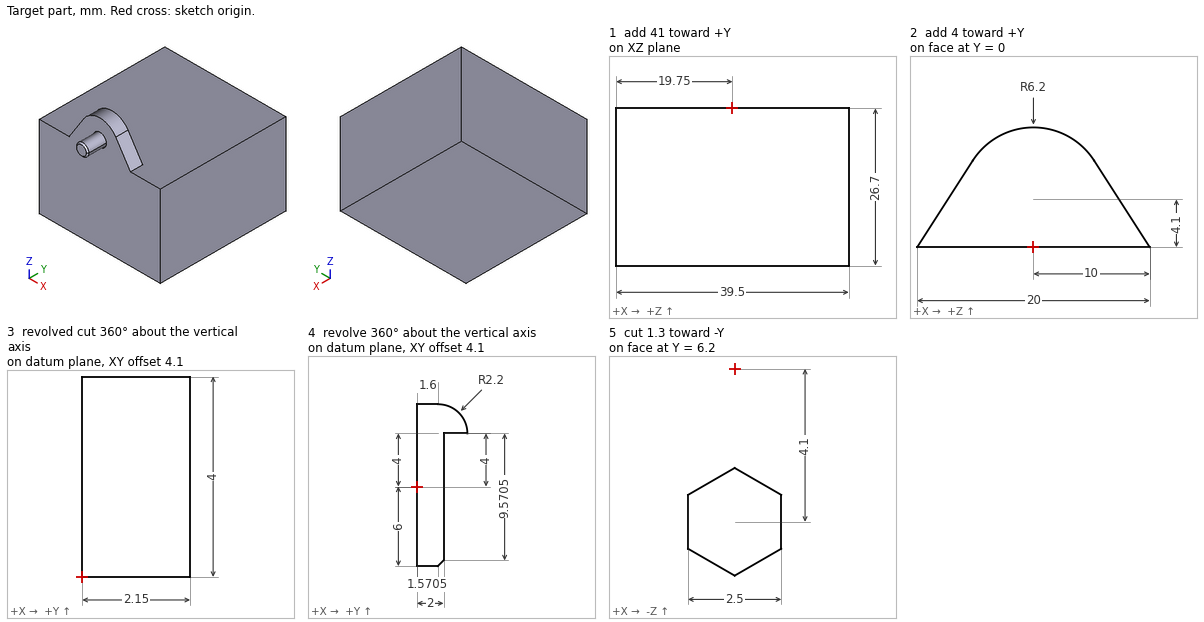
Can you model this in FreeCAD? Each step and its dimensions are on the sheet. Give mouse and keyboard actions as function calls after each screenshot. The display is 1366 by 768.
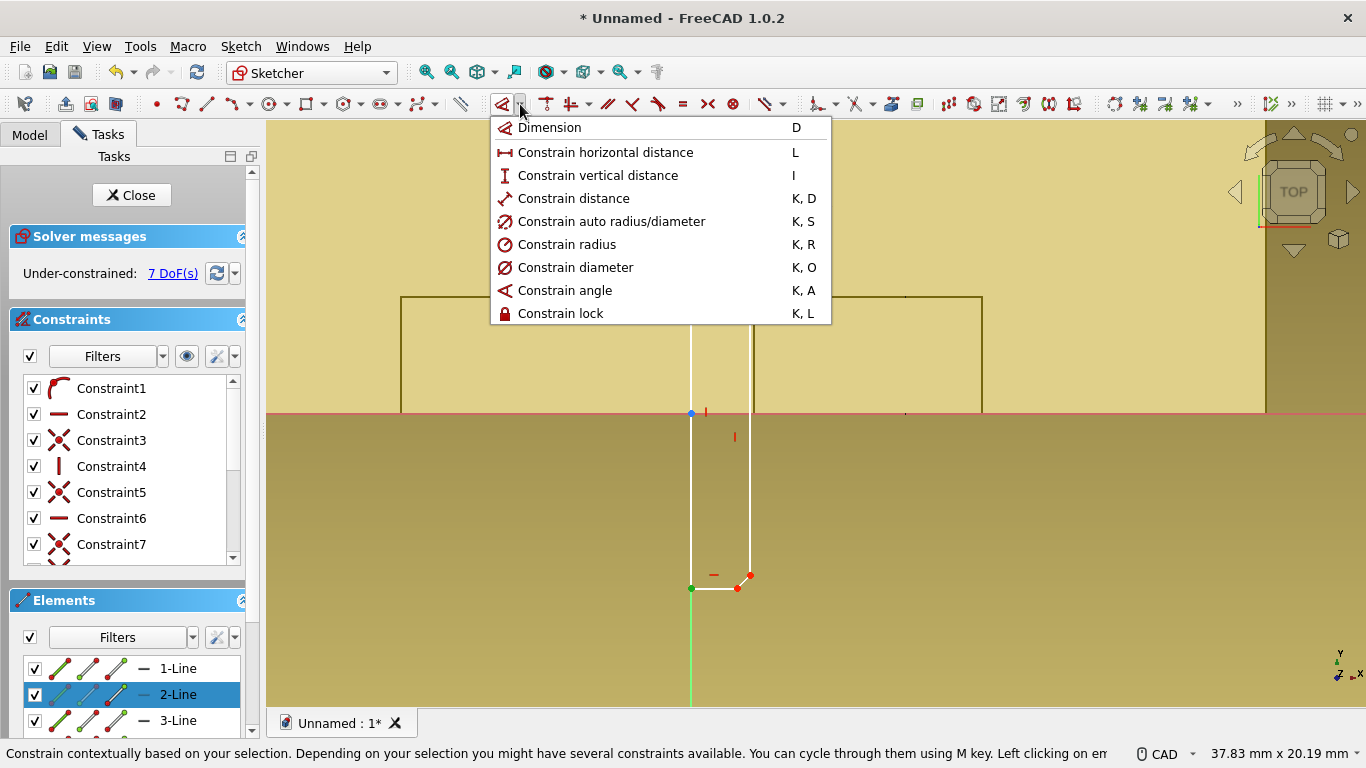
click(661, 176)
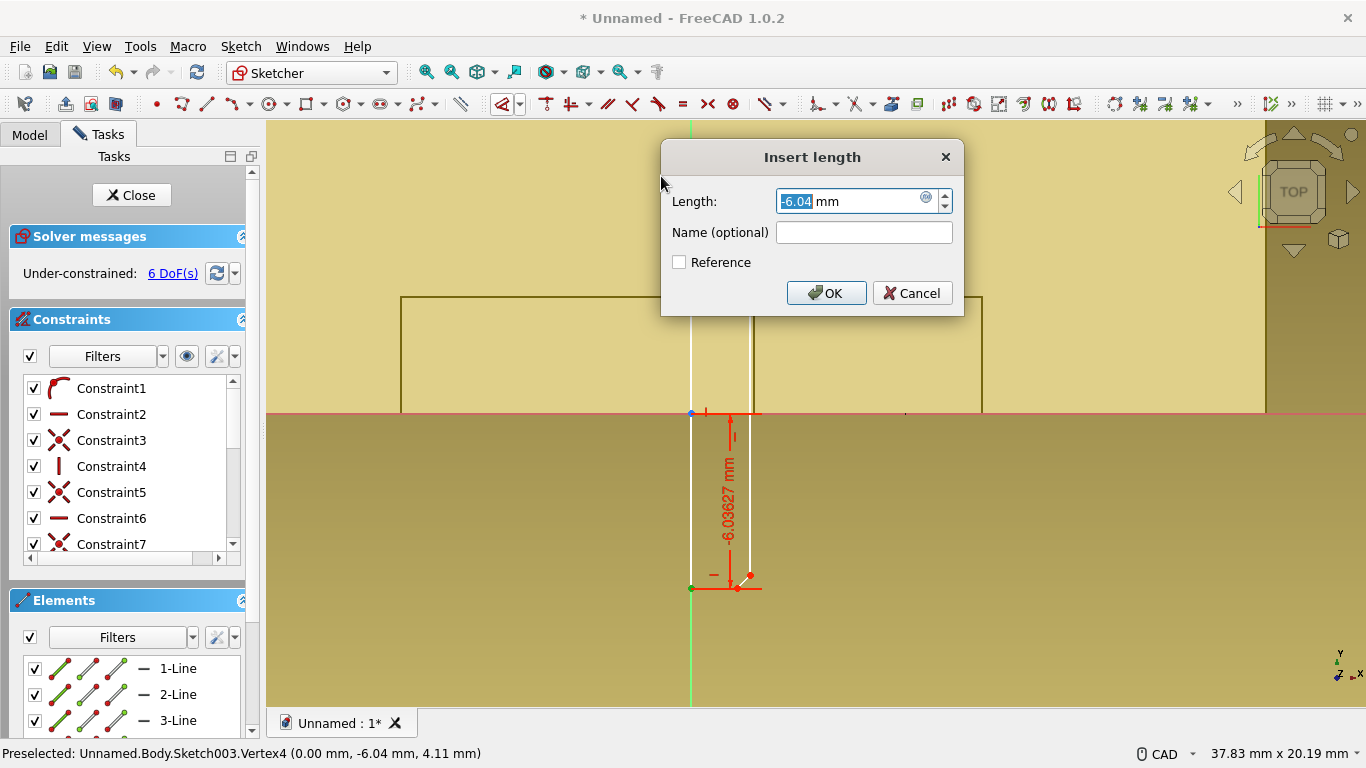
text(-6)
key(Return)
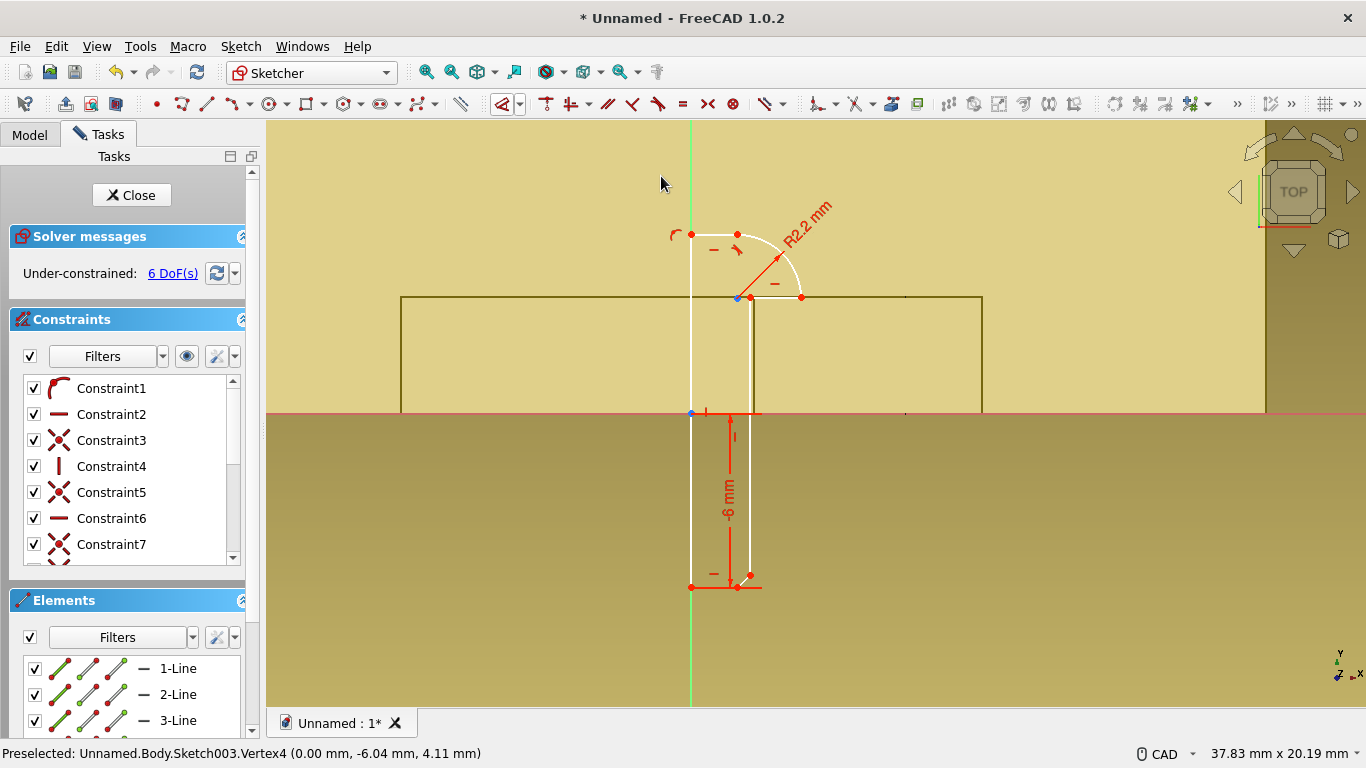
click(750, 576)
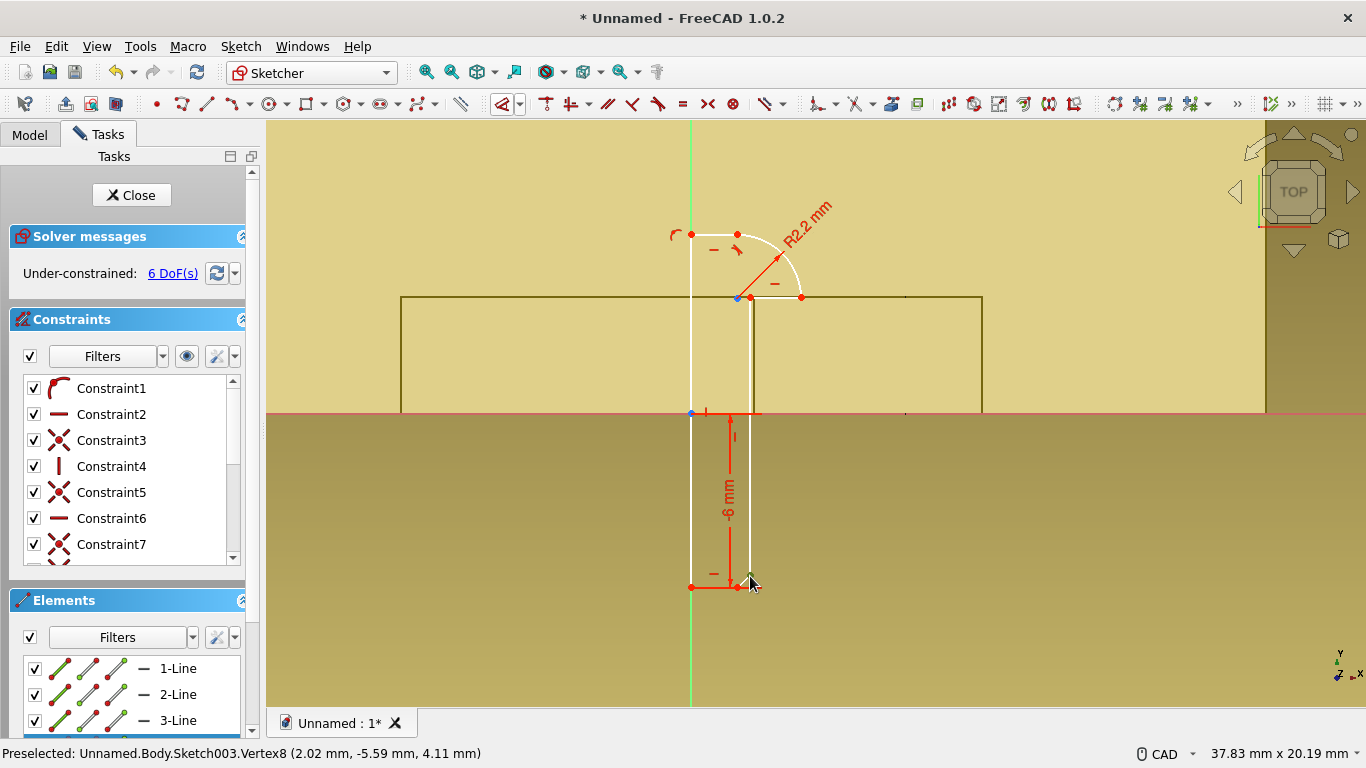
key(l)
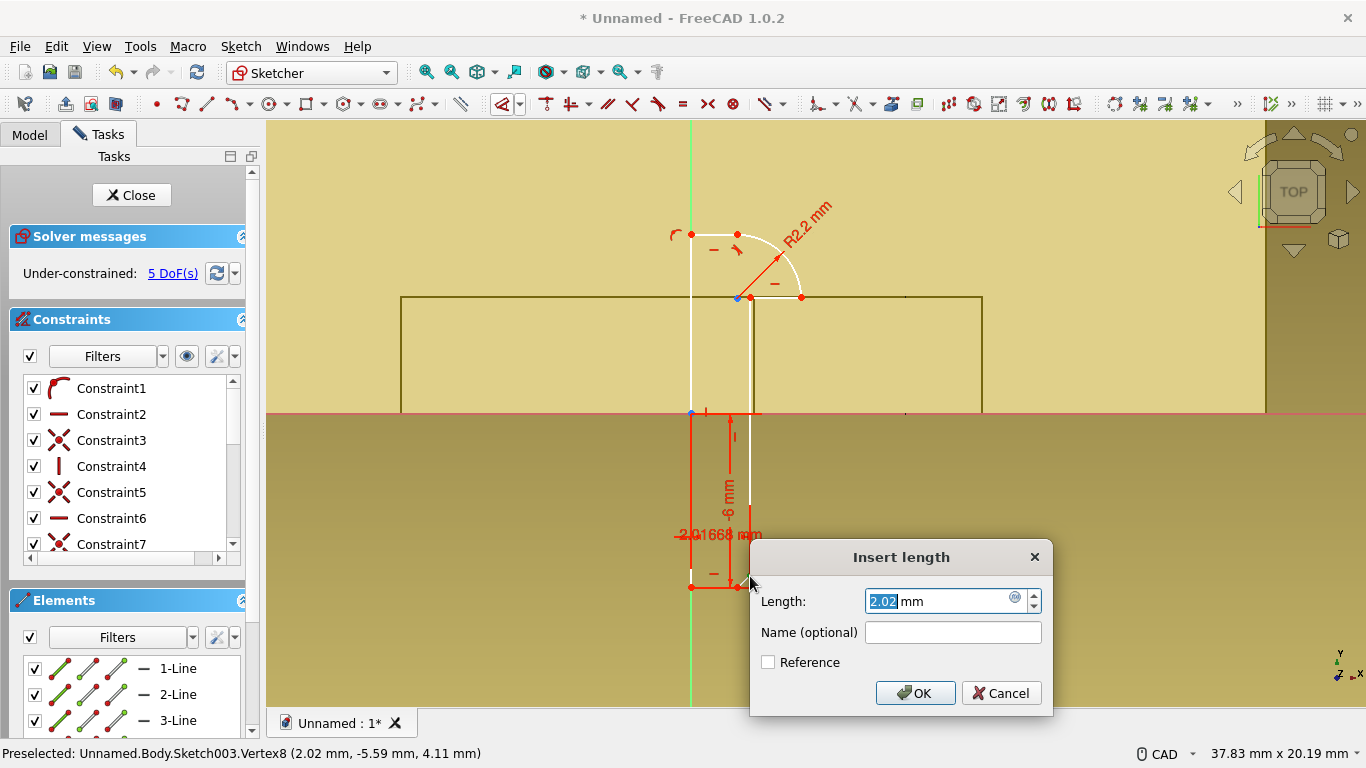
text(2)
key(Return)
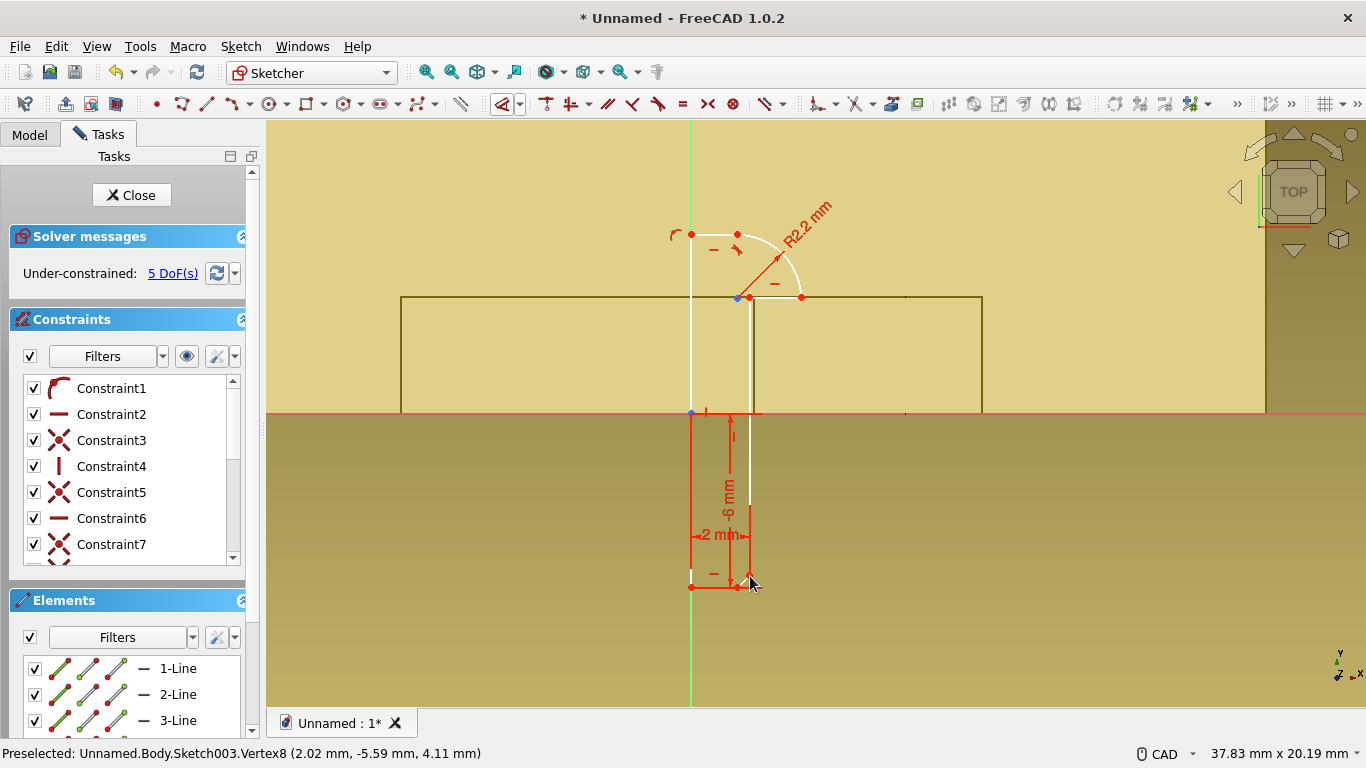
click(750, 298)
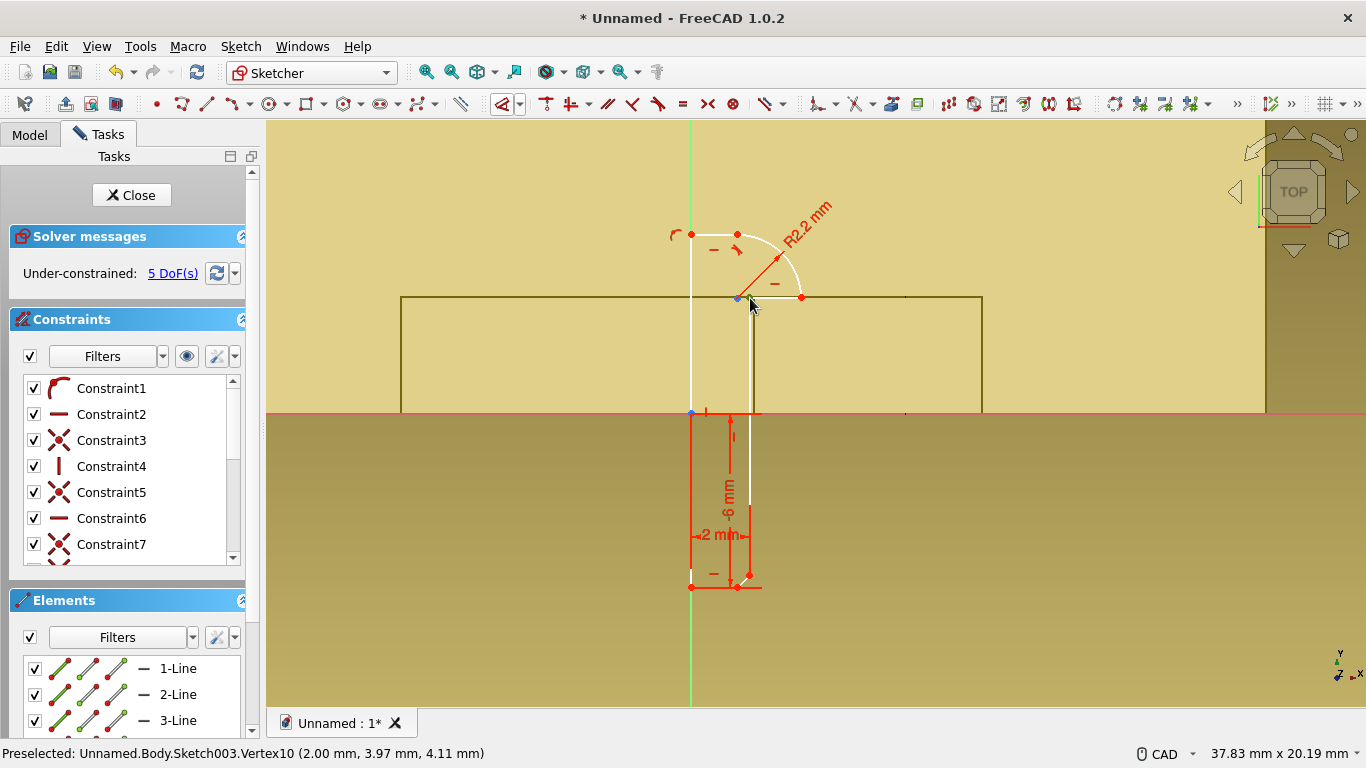
click(520, 104)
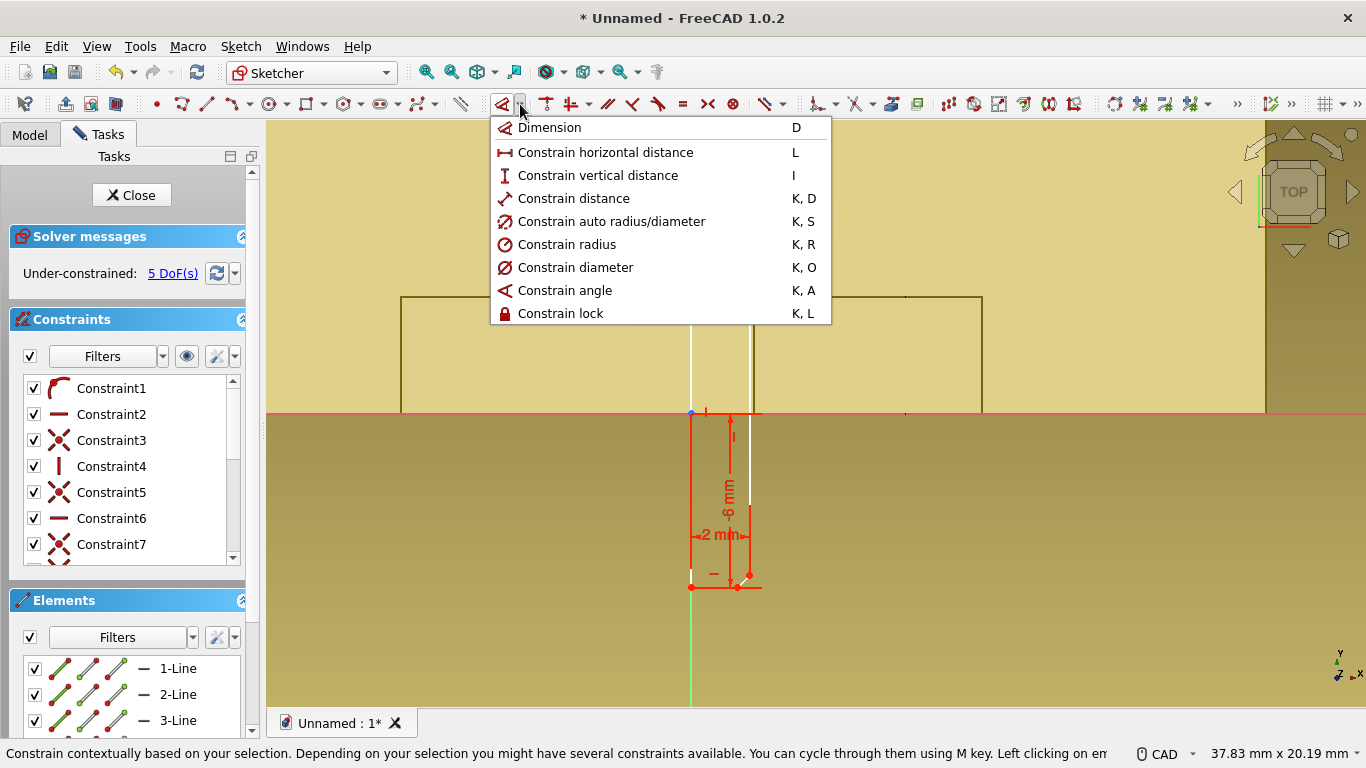
click(661, 176)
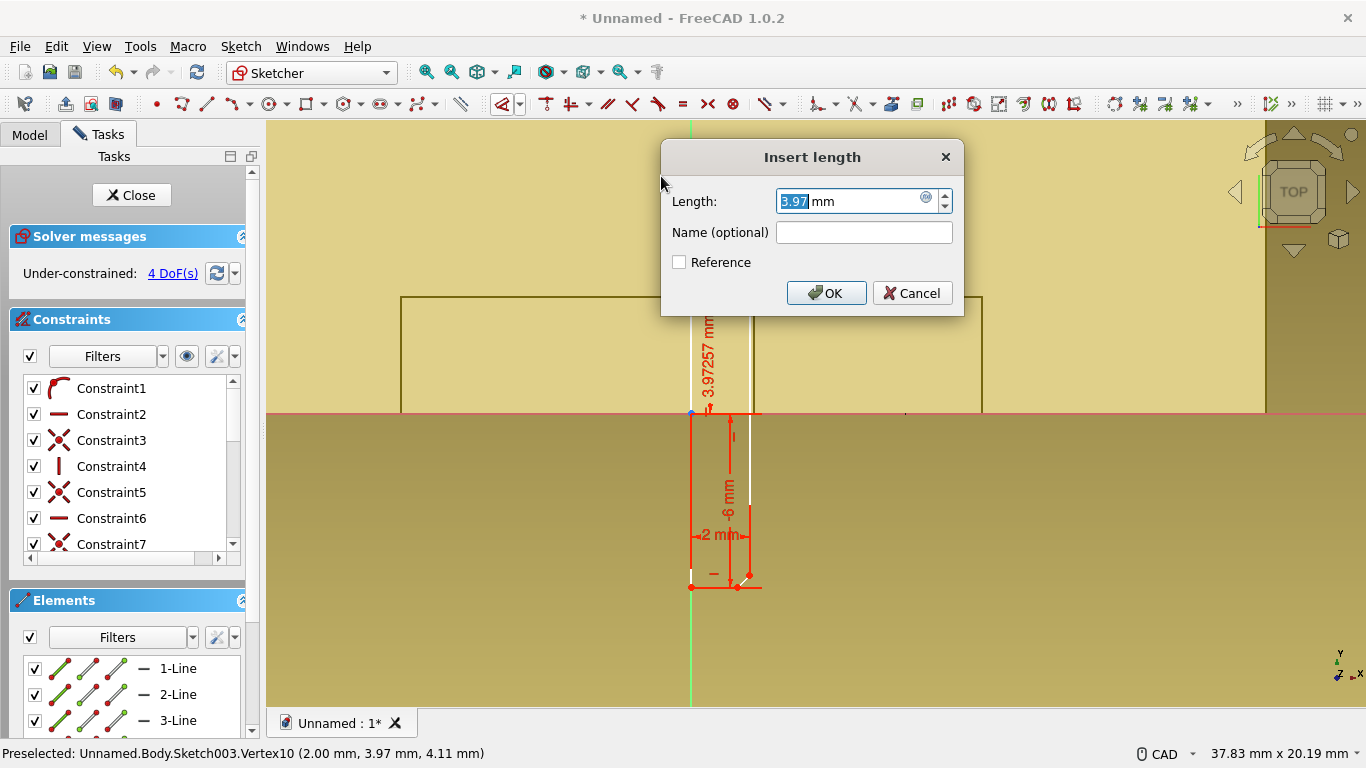
text(4)
key(Return)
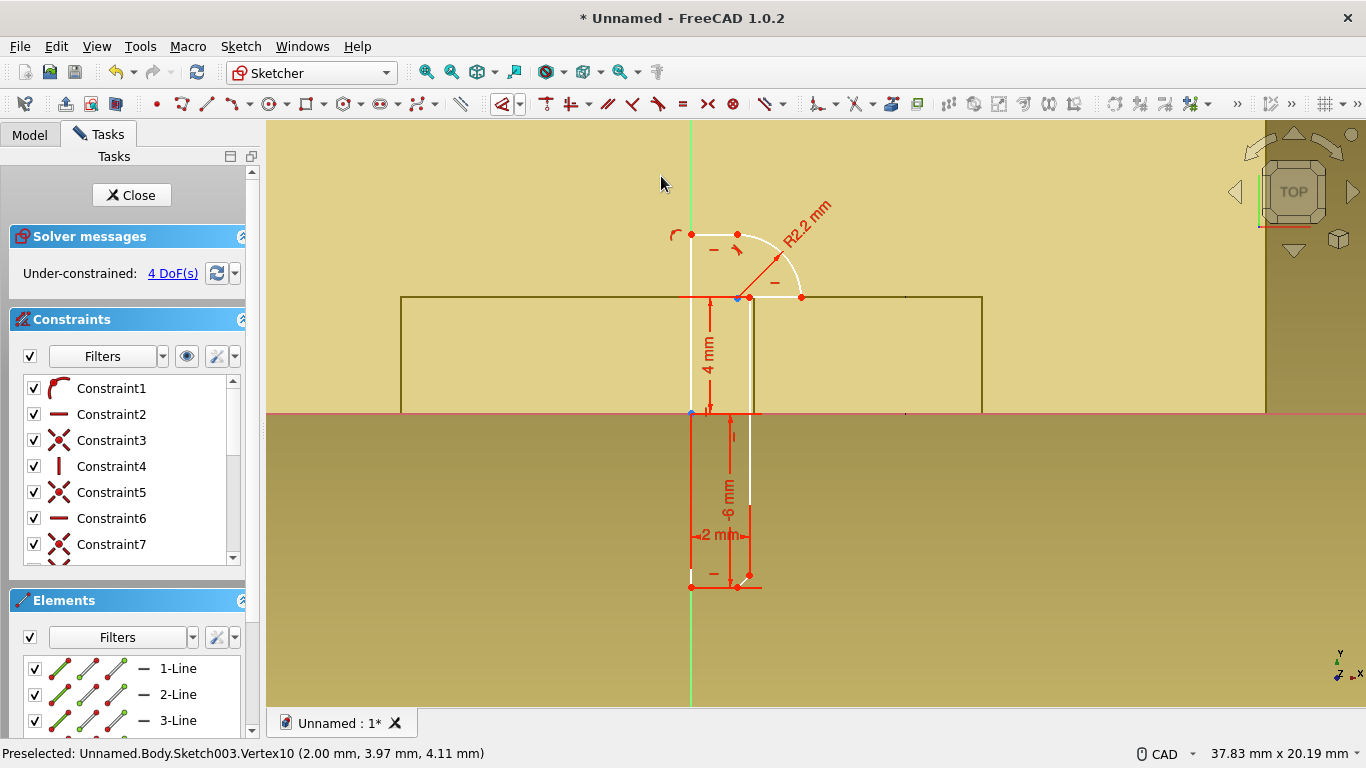
click(737, 299)